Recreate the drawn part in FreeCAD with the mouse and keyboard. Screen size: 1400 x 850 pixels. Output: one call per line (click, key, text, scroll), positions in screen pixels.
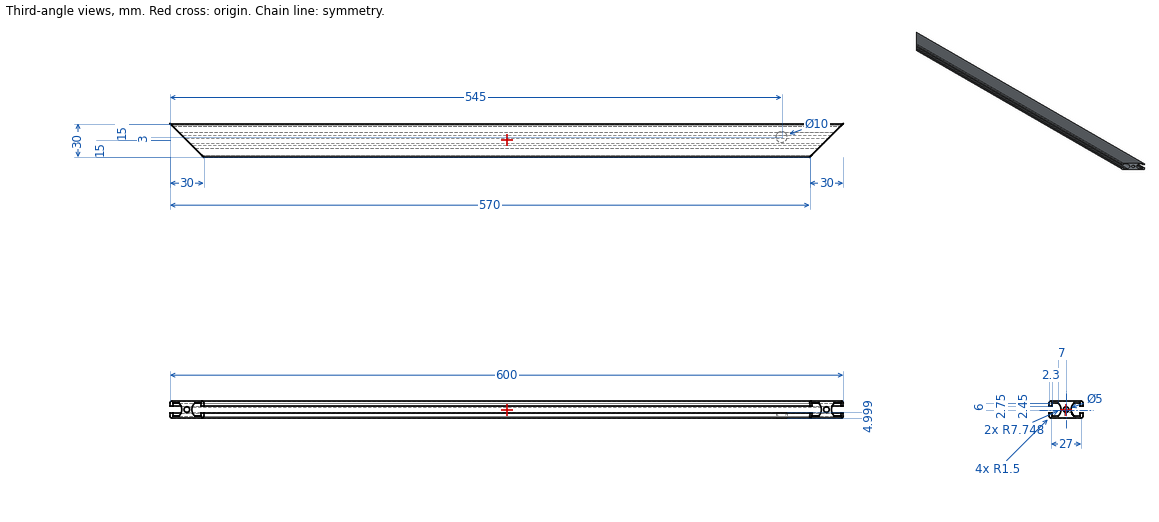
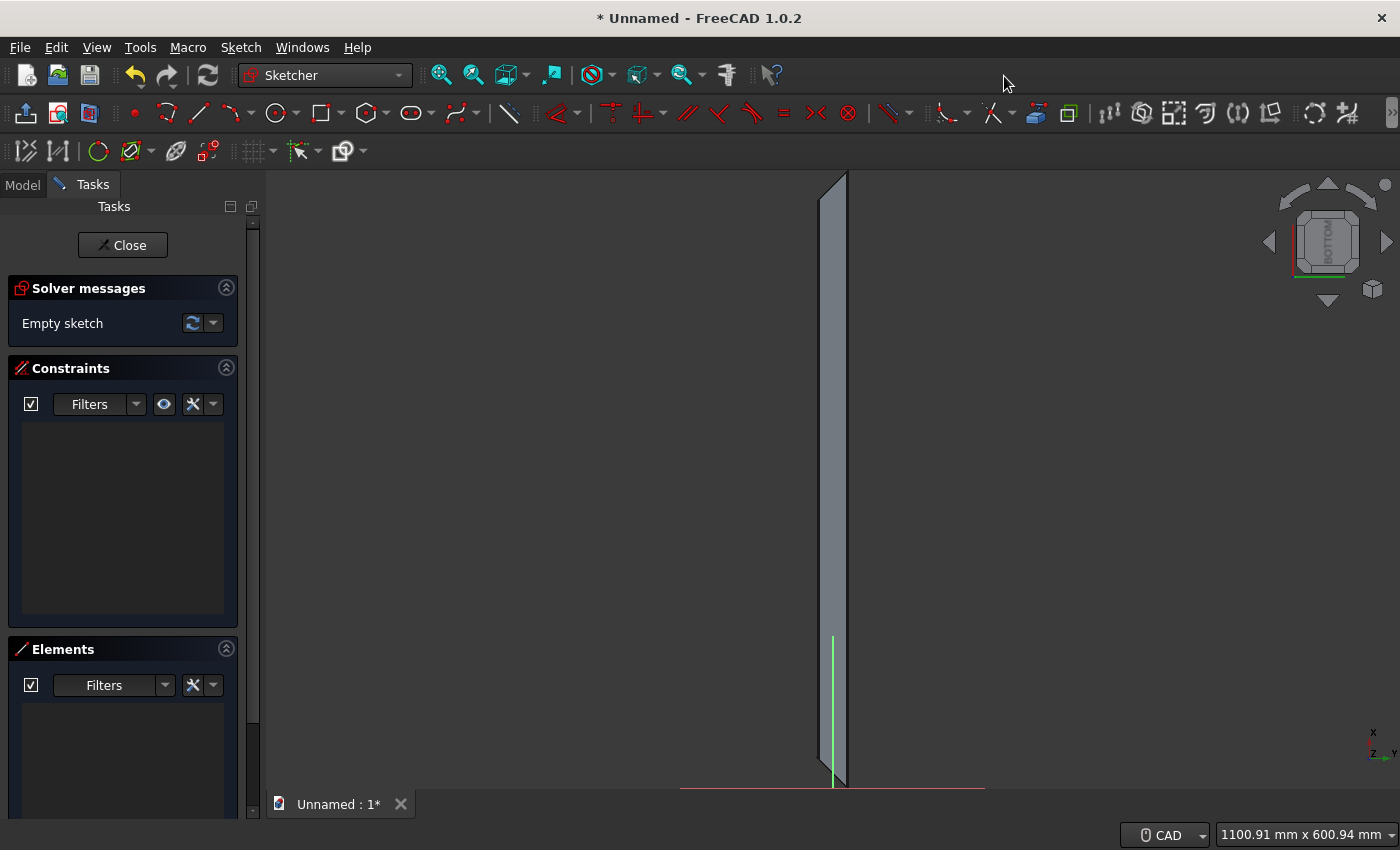
scroll(840, 214, up, 15)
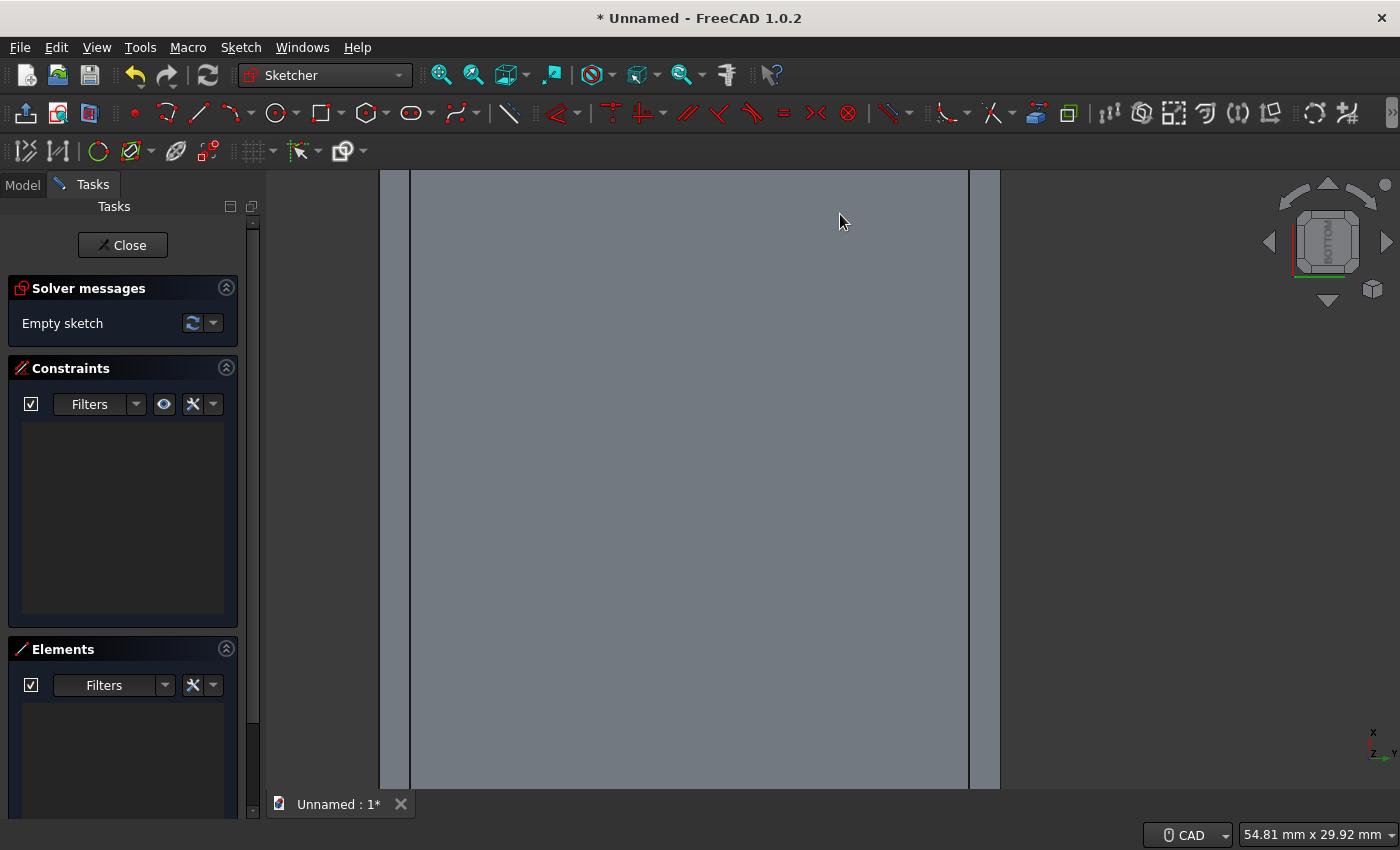
scroll(736, 473, up, 3)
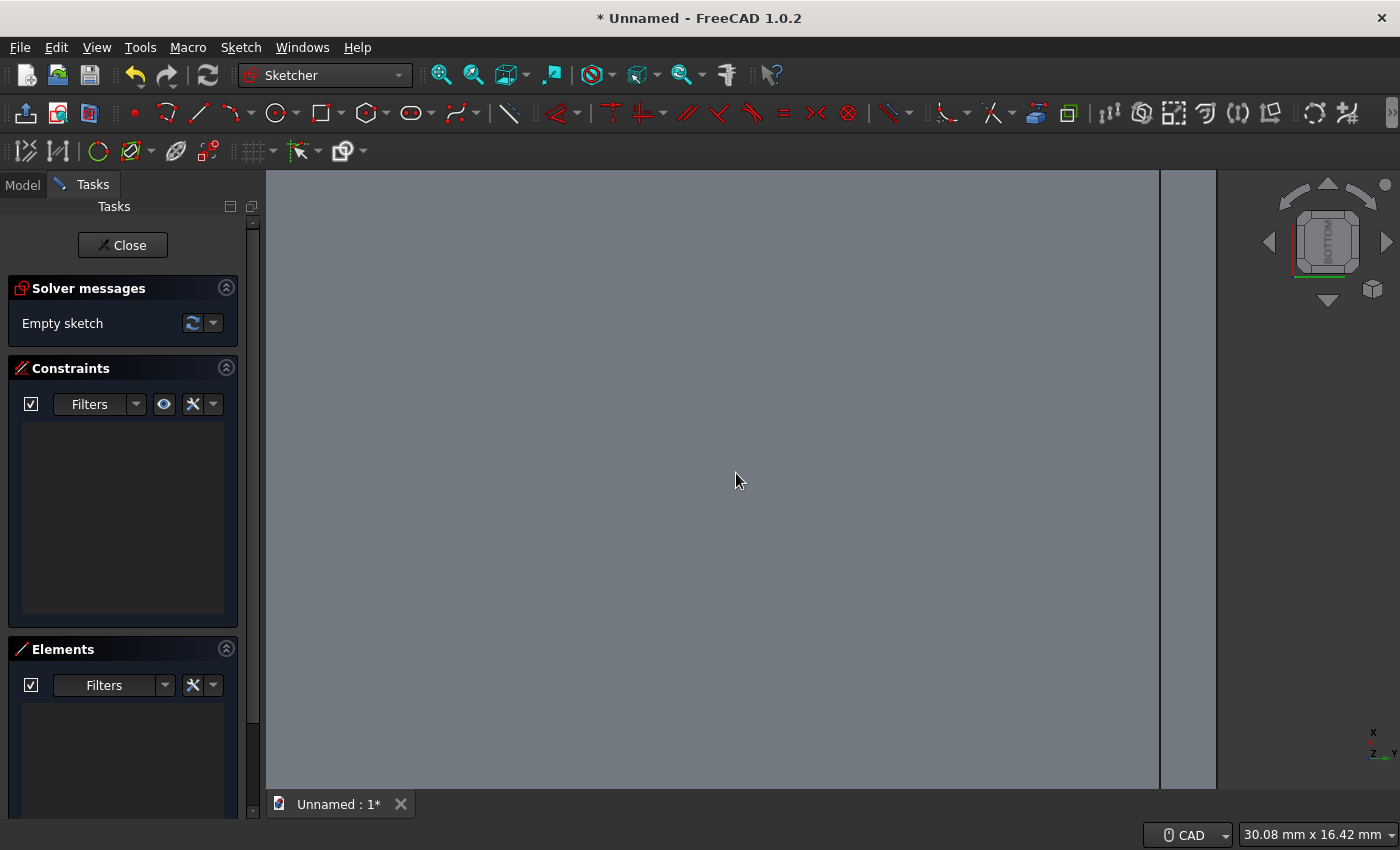
key(g)
key(c)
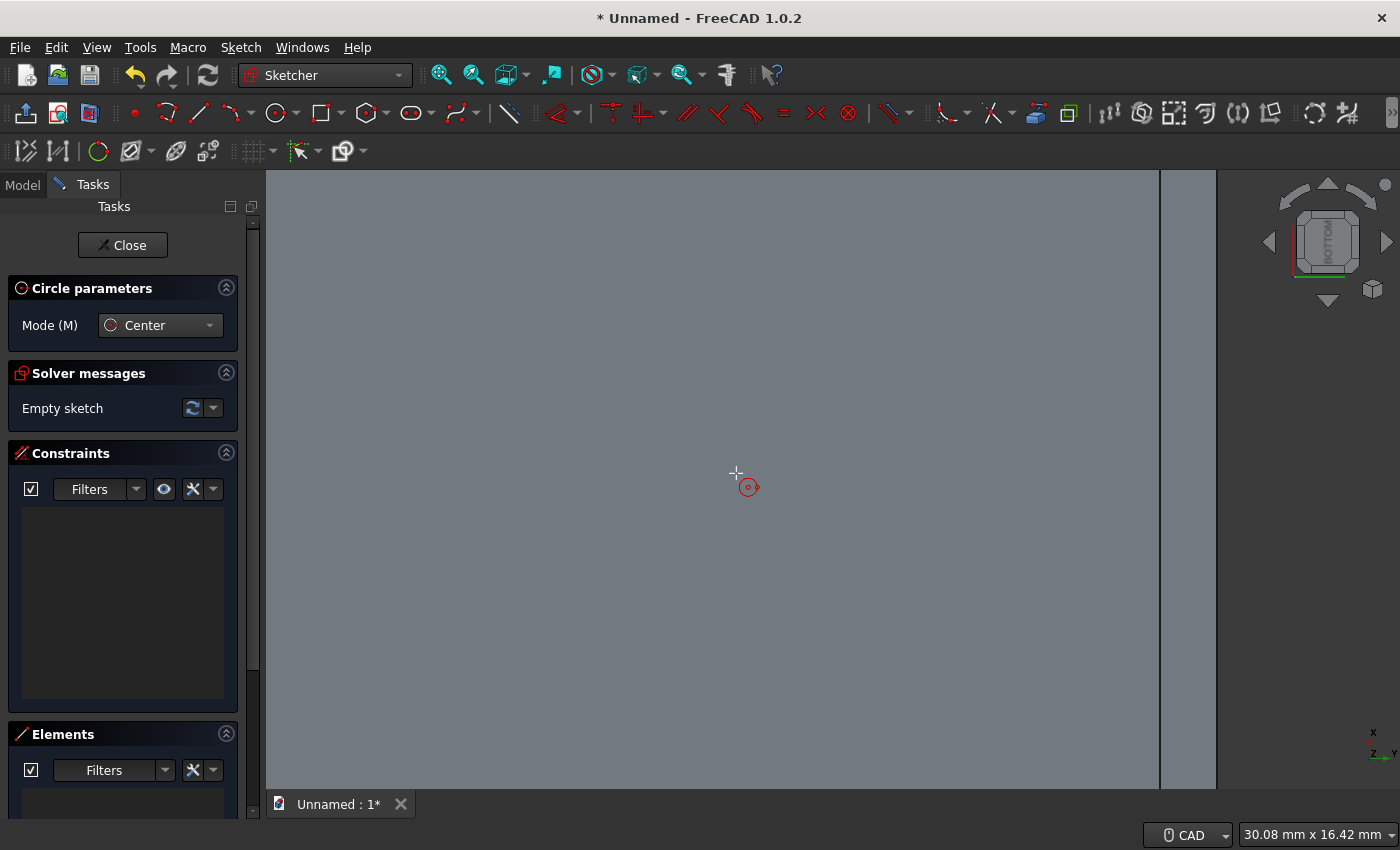
click(764, 479)
move(898, 346)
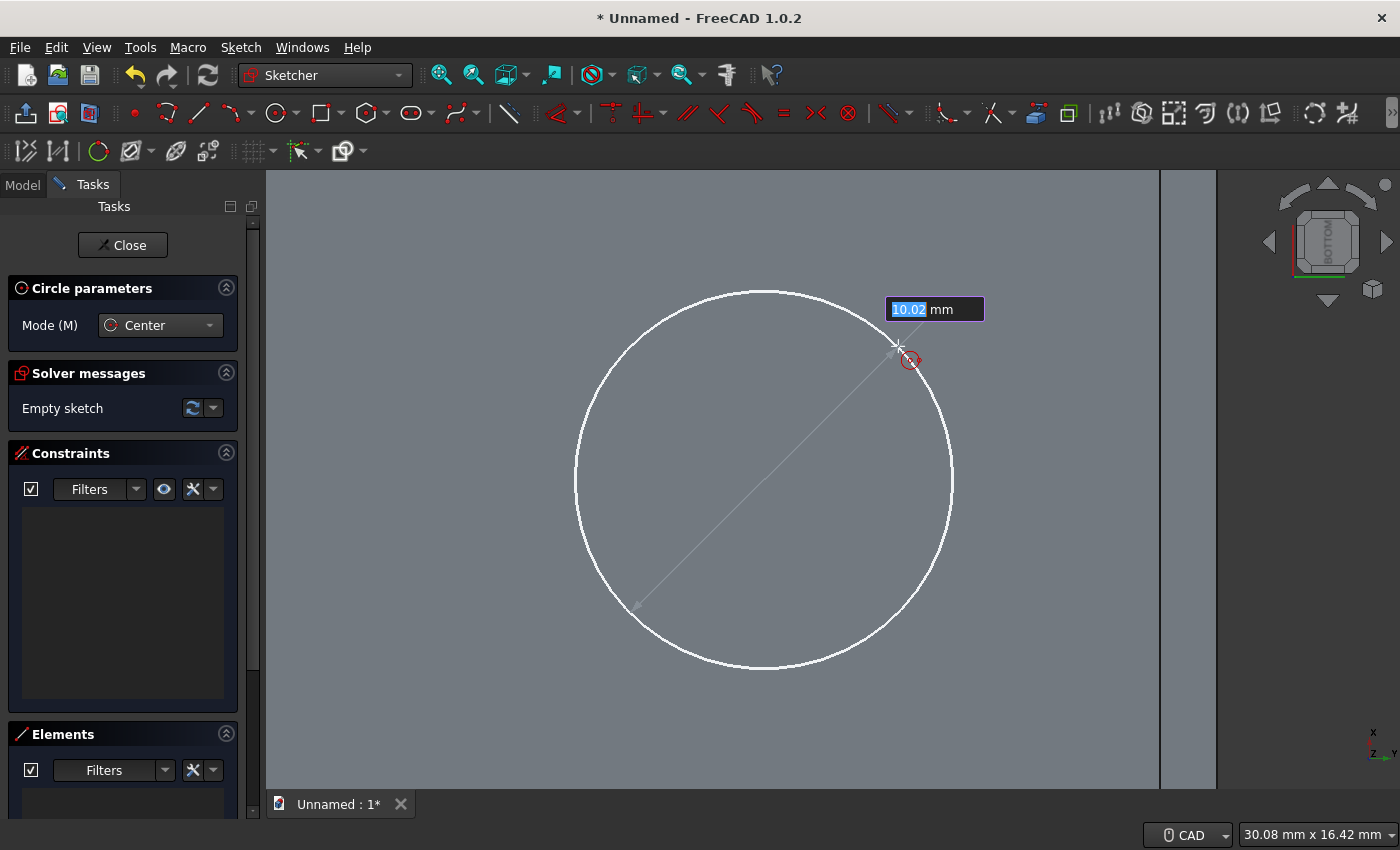
text(10)
key(Return)
key(Escape)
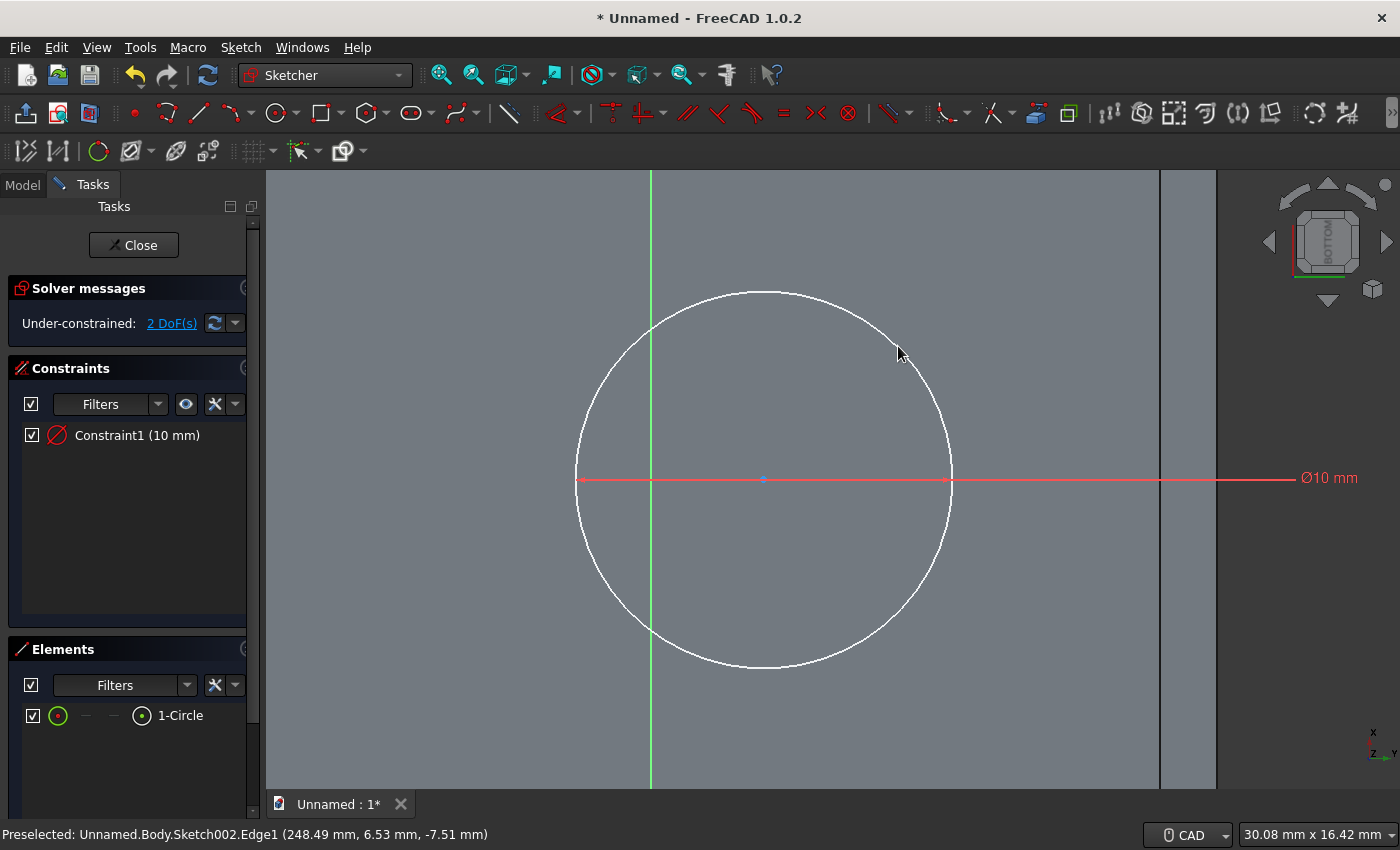
click(556, 114)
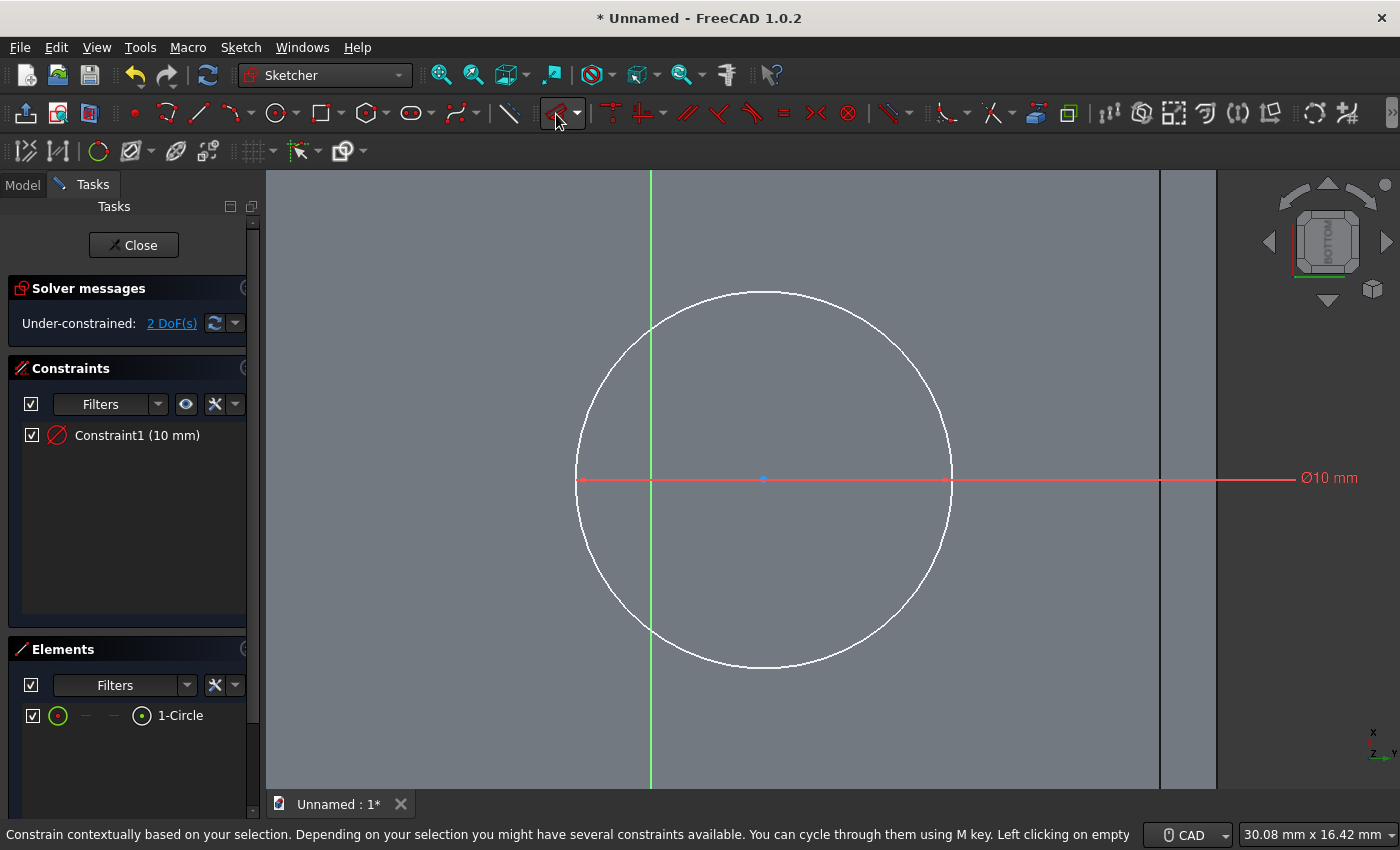
click(764, 480)
click(708, 446)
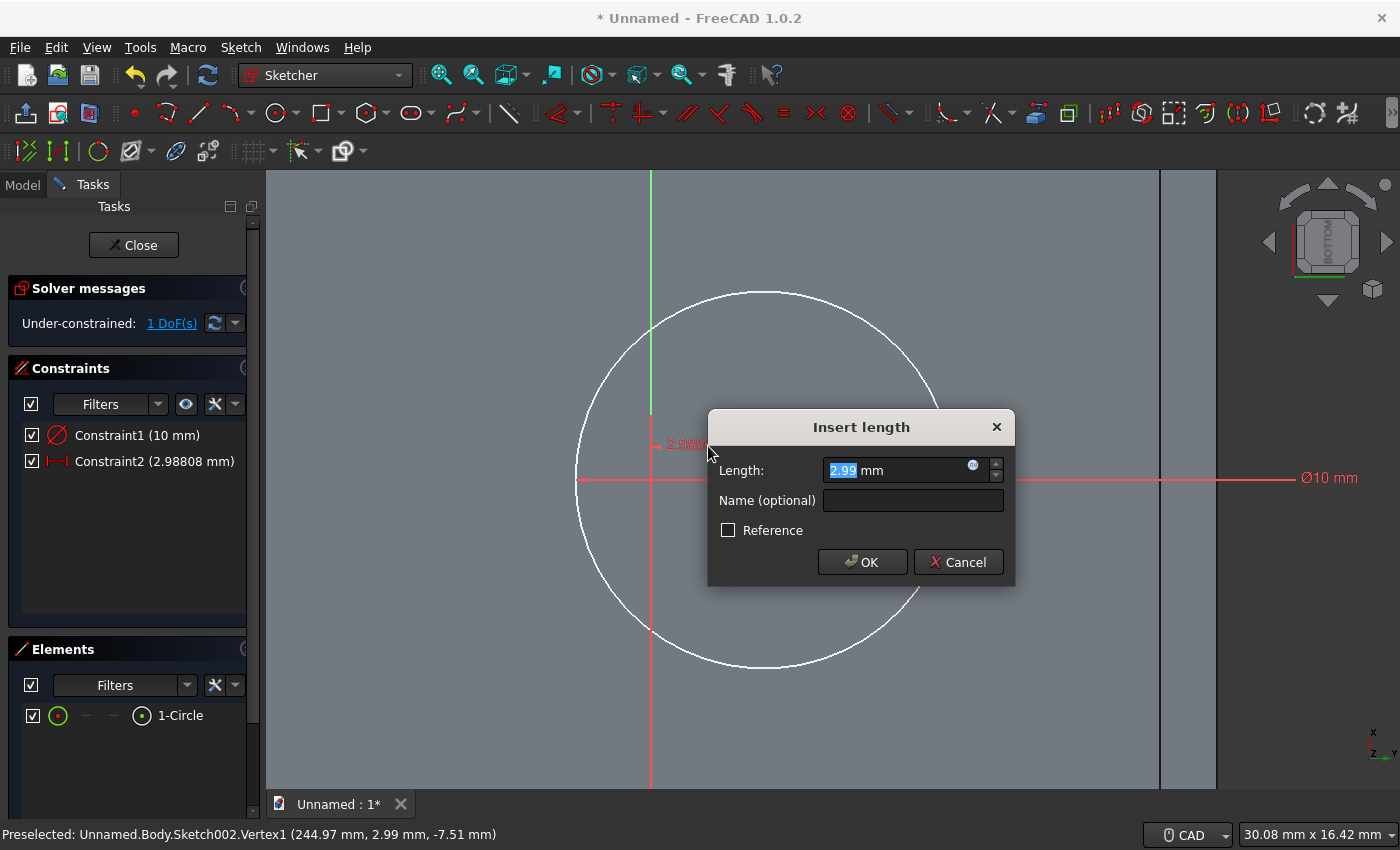
text(3)
key(Return)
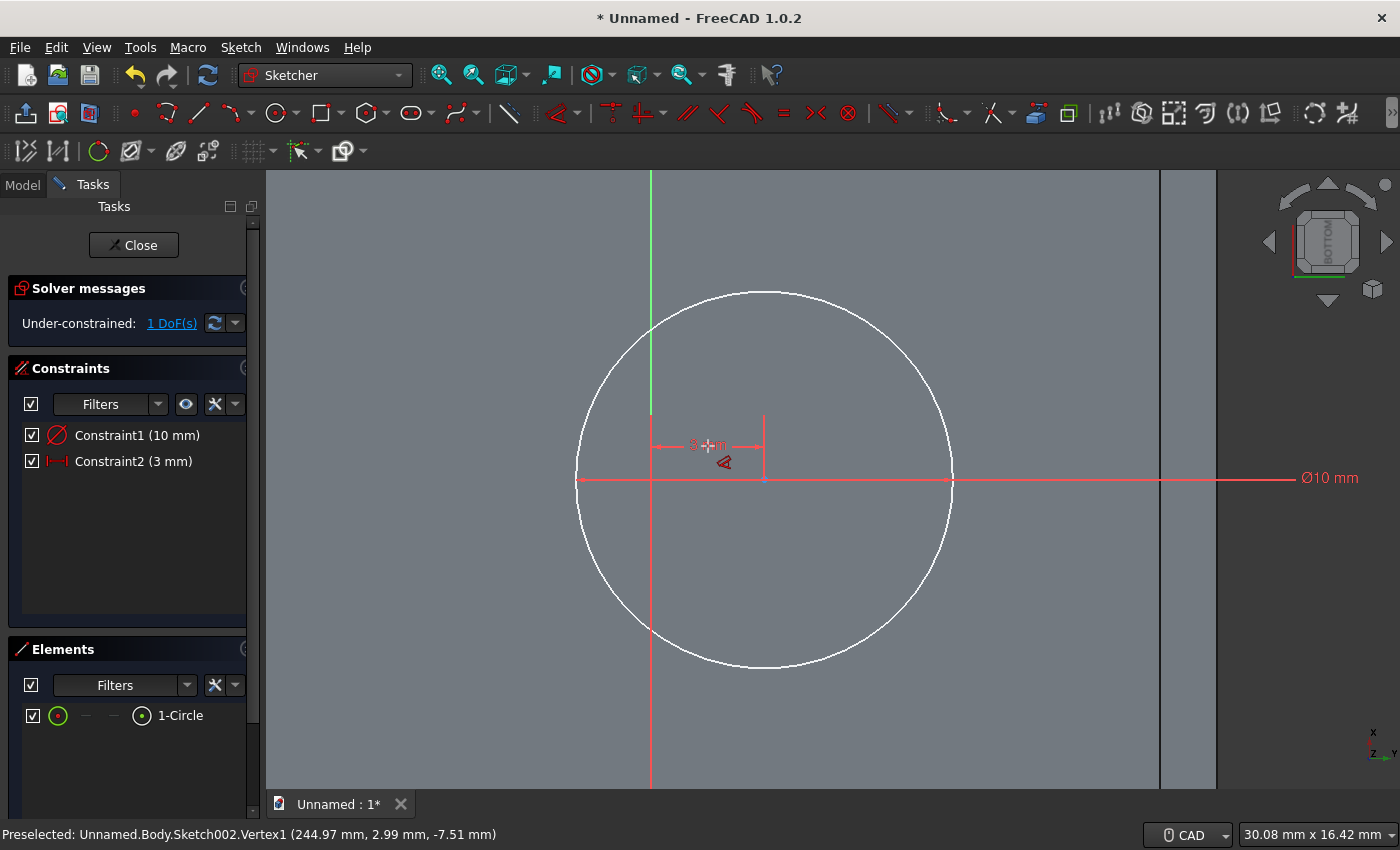
click(764, 480)
click(617, 620)